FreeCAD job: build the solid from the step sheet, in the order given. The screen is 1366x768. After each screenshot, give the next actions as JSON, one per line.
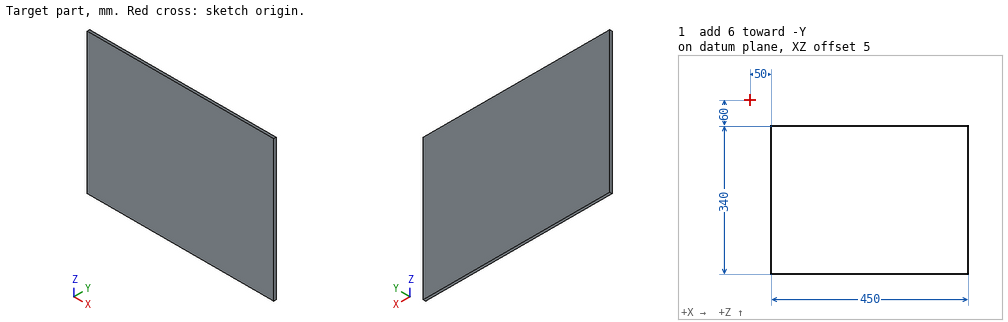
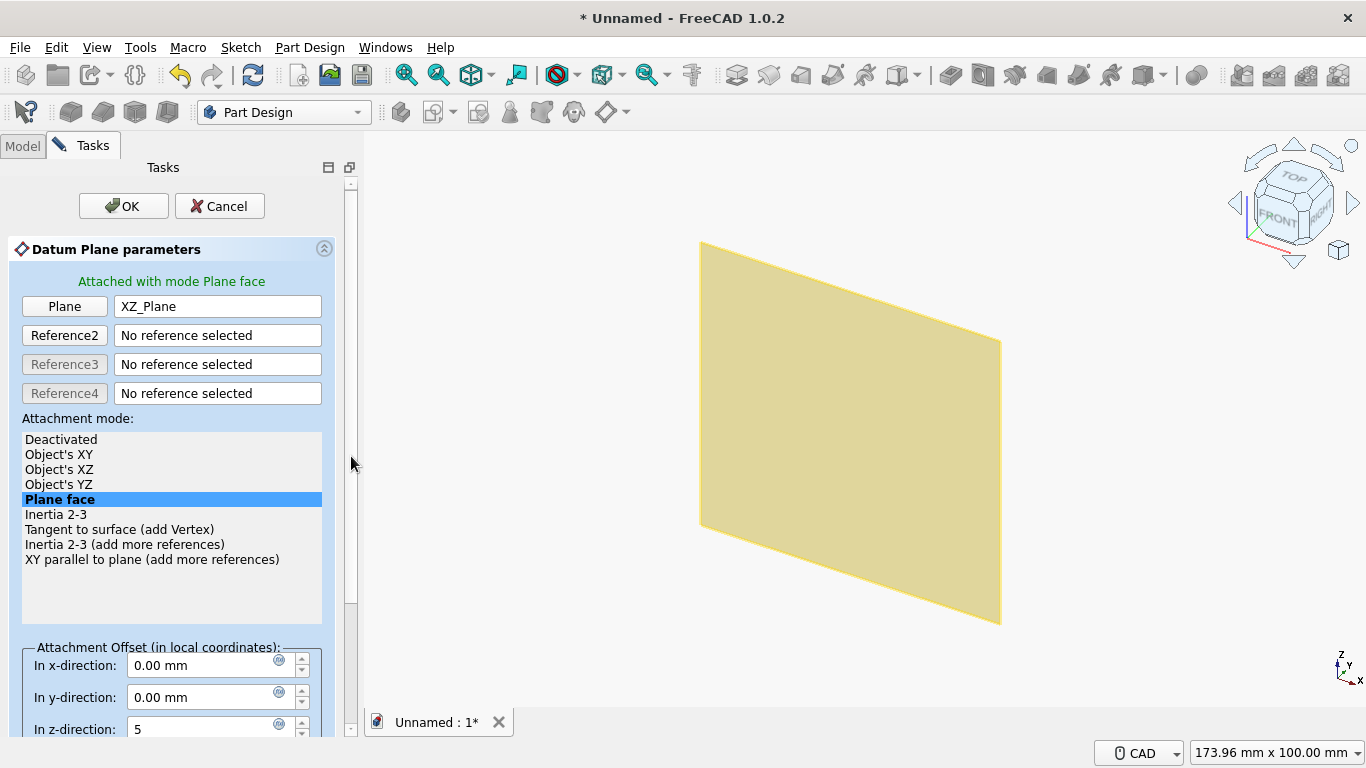
{"action": "left_click", "coordinate": [124, 206]}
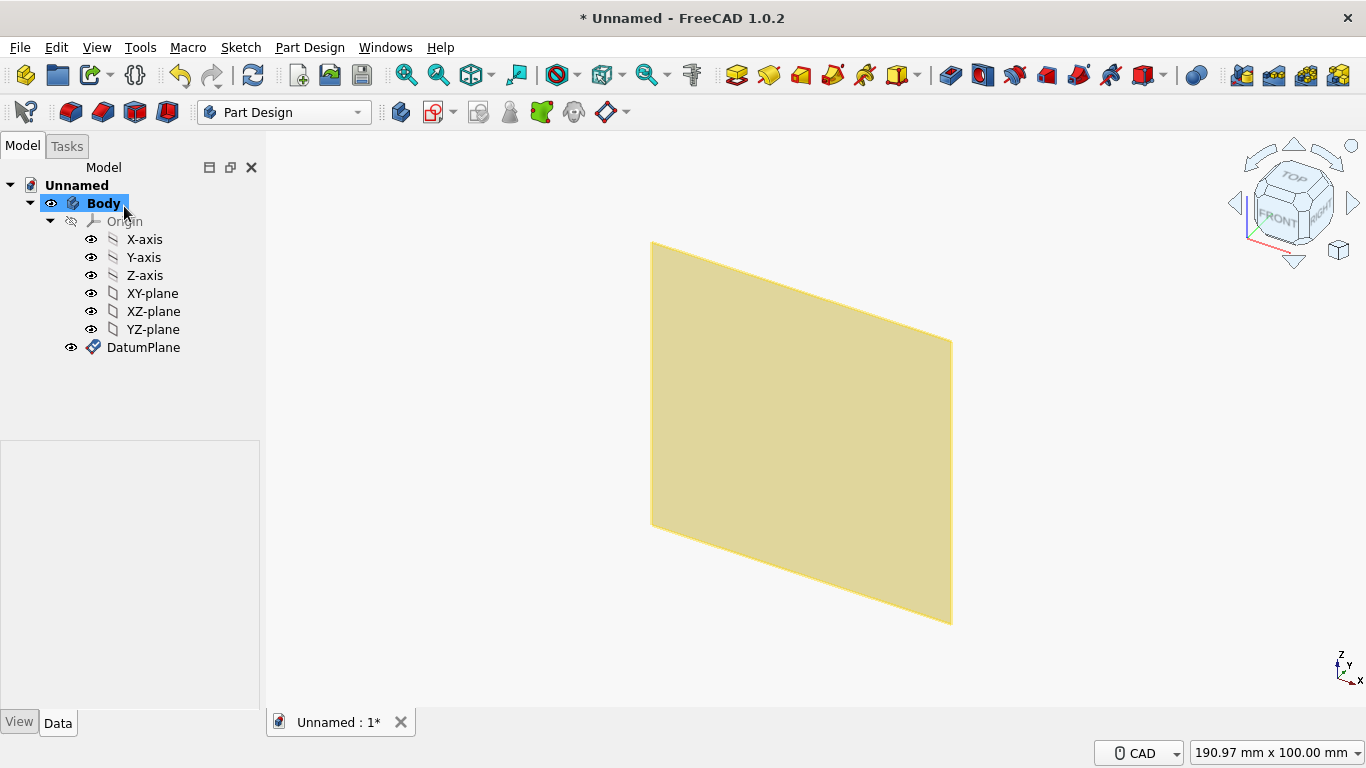
{"action": "left_click", "coordinate": [116, 347]}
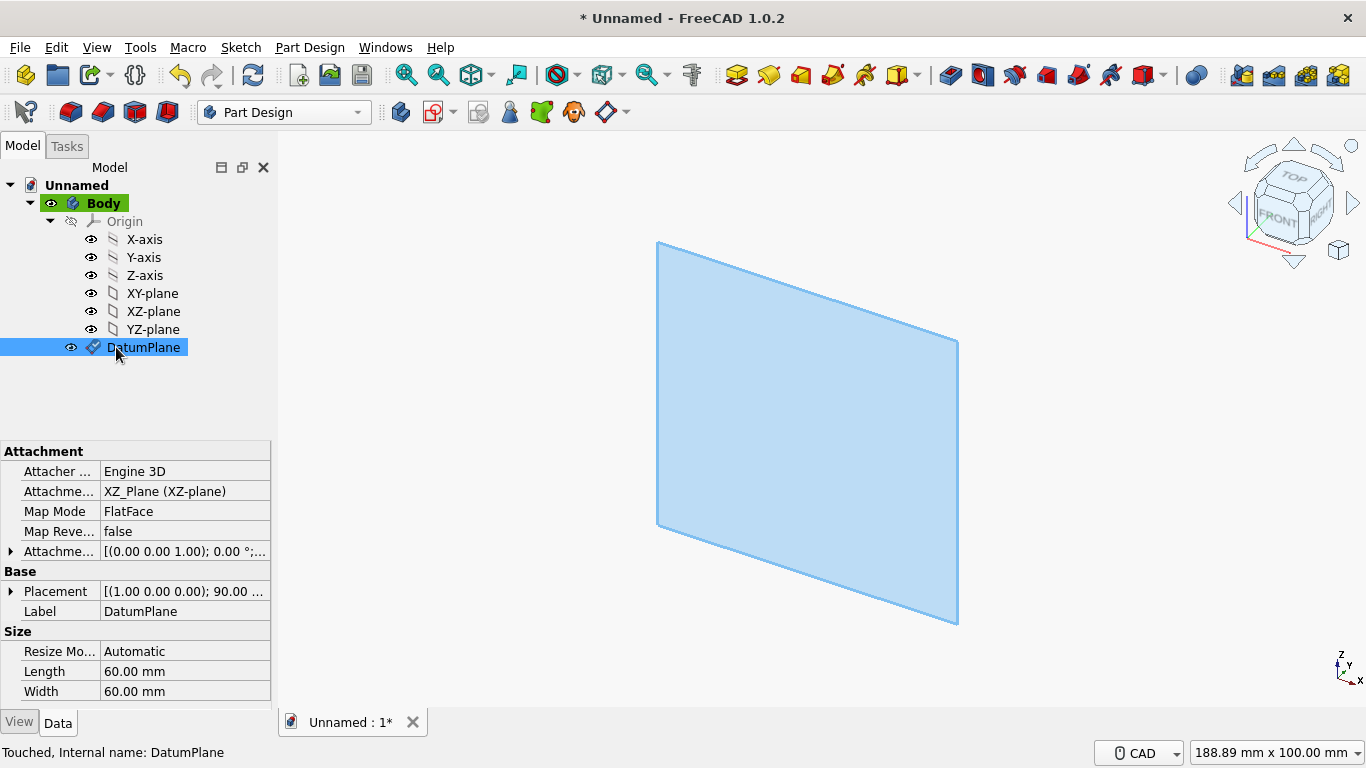
{"action": "left_click", "coordinate": [434, 112]}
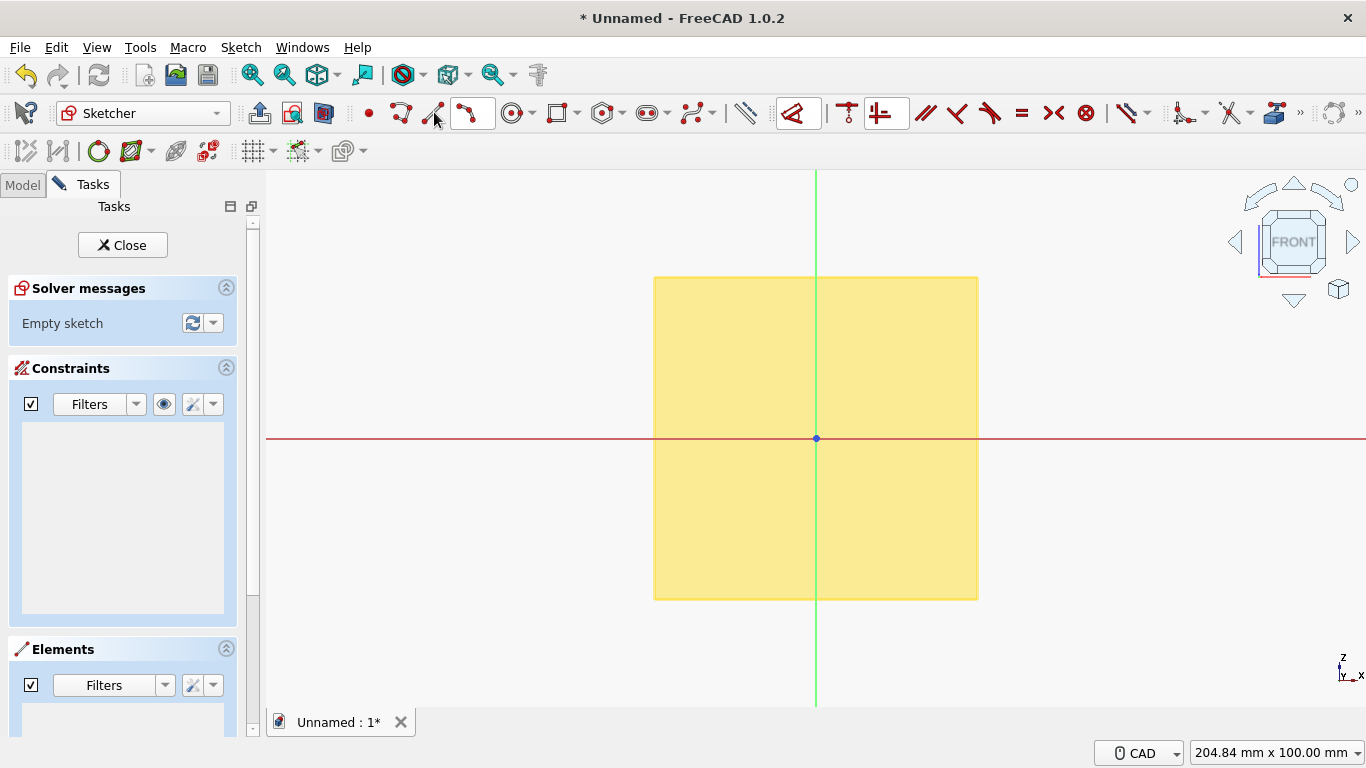
{"action": "scroll", "coordinate": [468, 226], "scroll_direction": "down", "scroll_amount": 9}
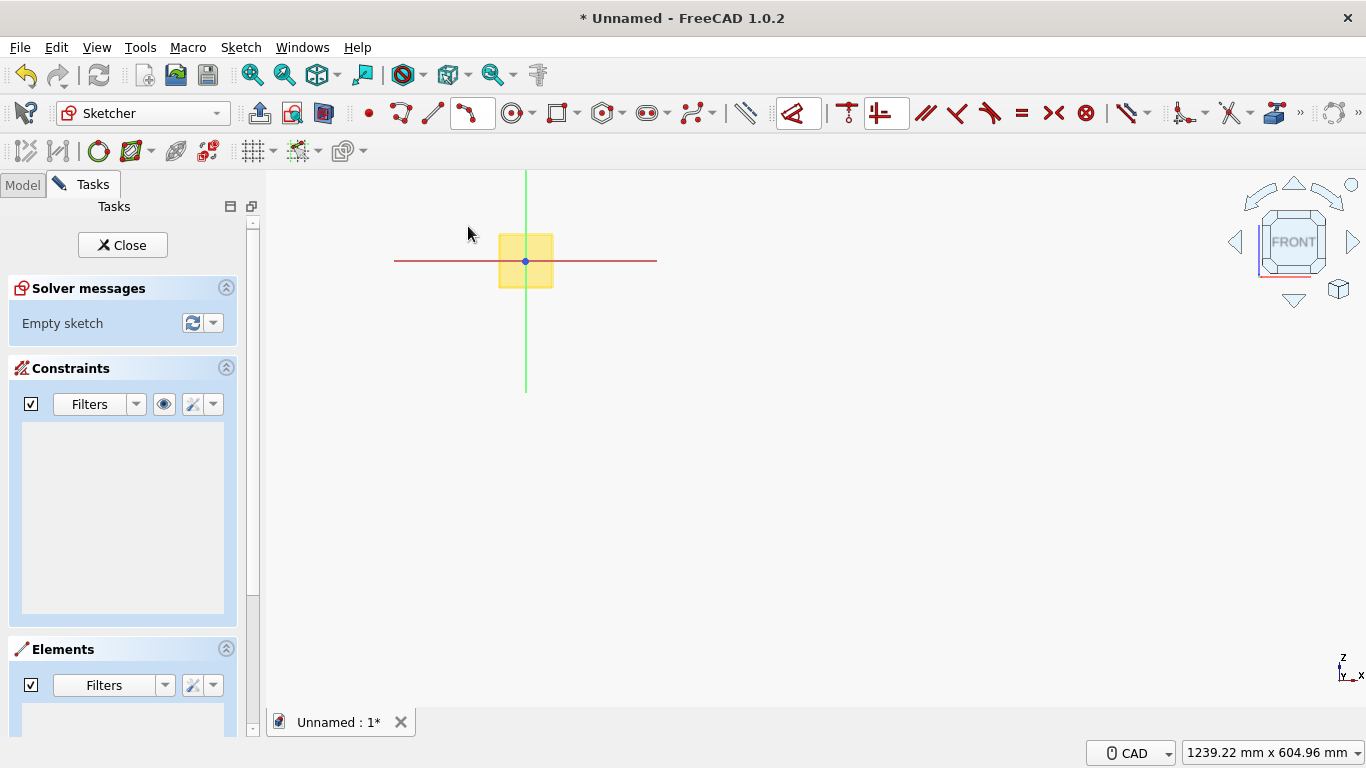
{"action": "key", "text": "g r"}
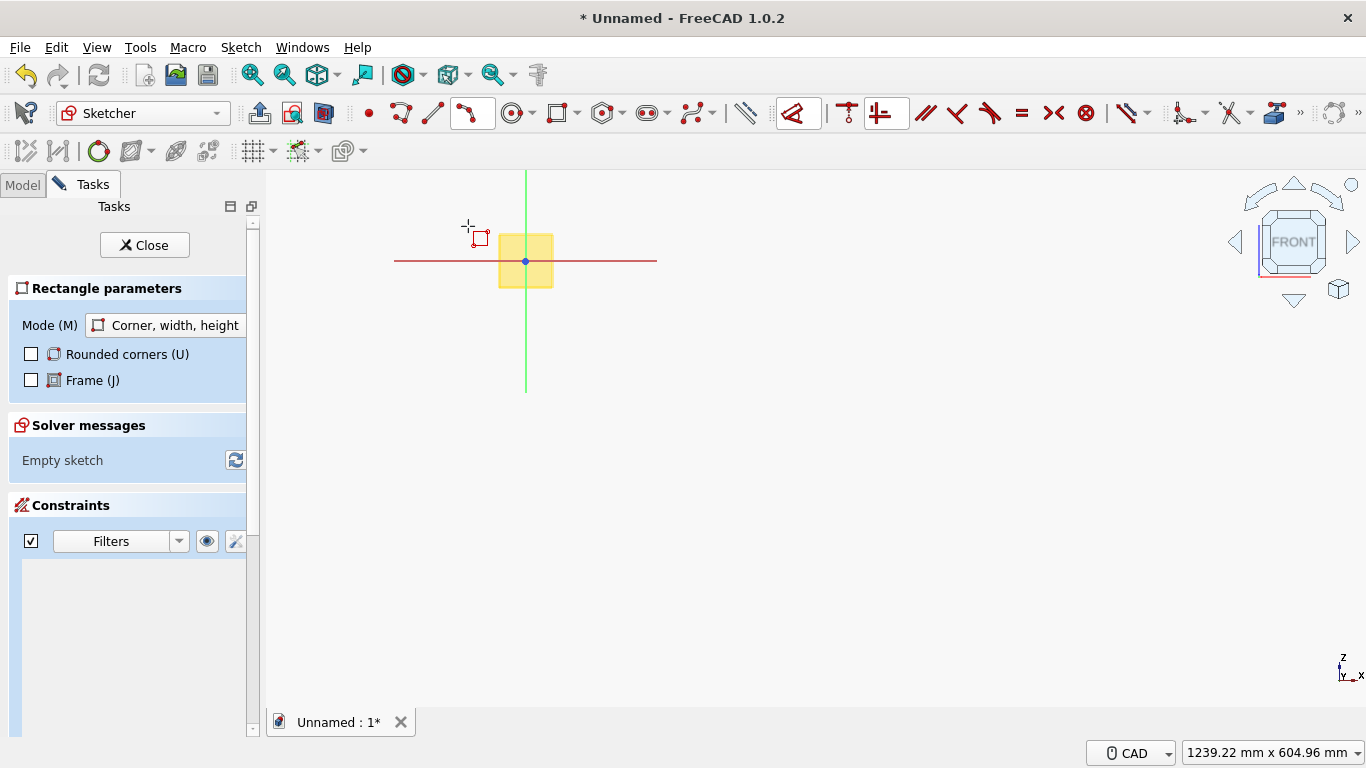
{"action": "left_click", "coordinate": [570, 314]}
{"action": "left_click", "coordinate": [970, 616]}
{"action": "key", "text": "Escape"}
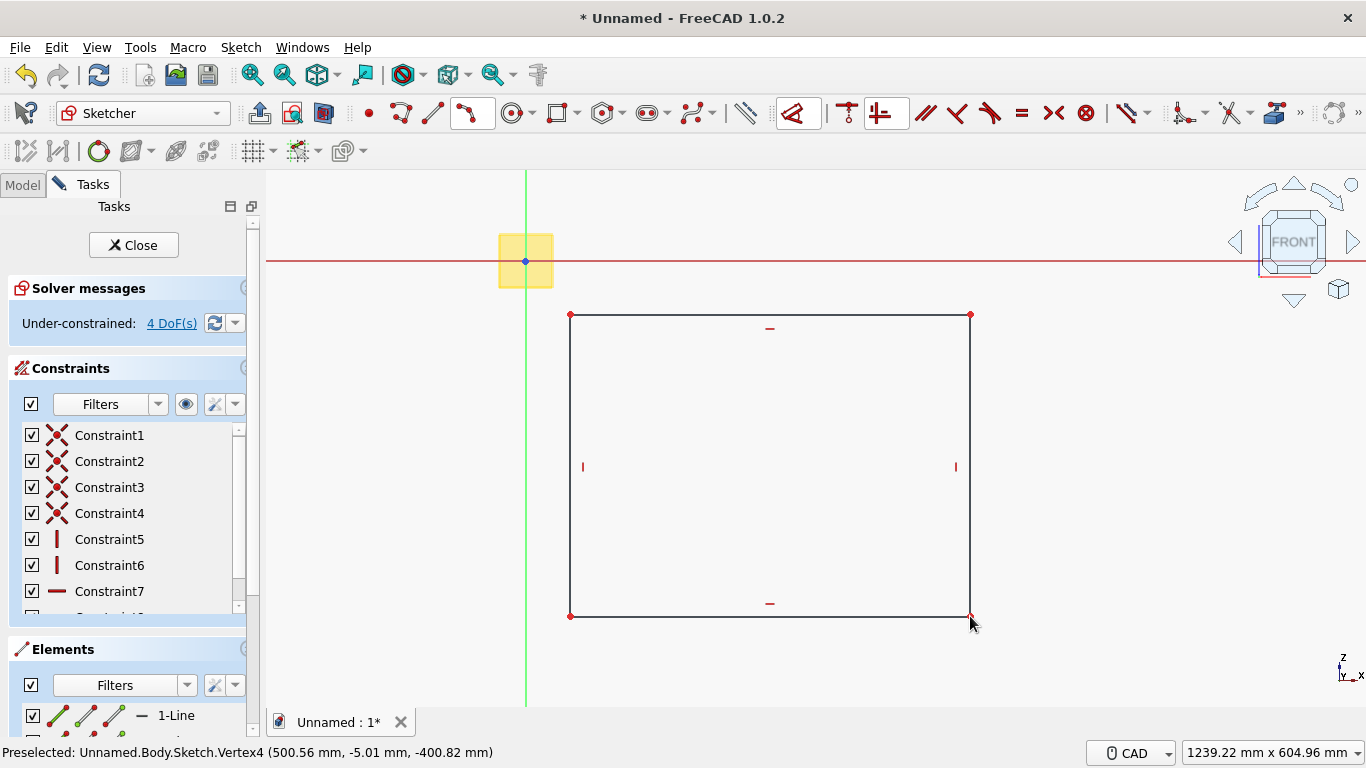
{"action": "key", "text": "d"}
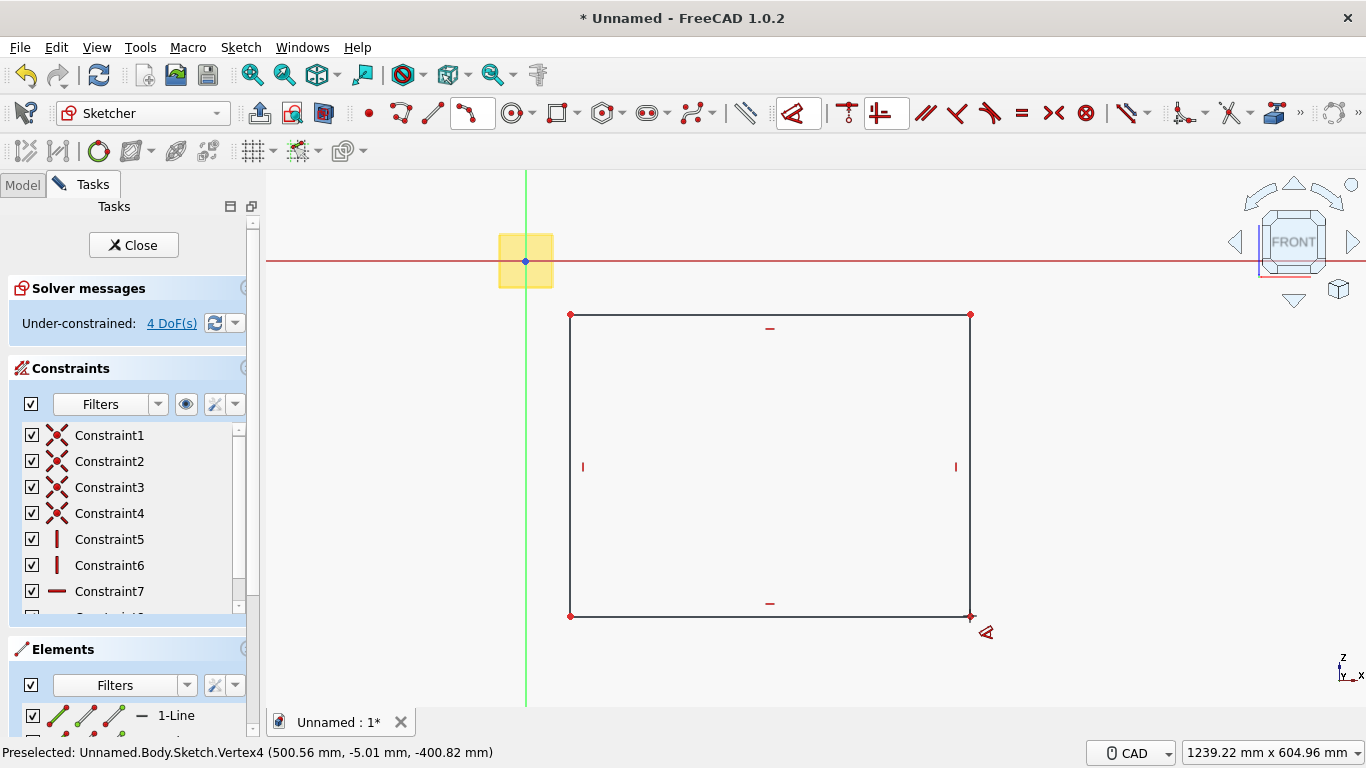
{"action": "left_click", "coordinate": [570, 406]}
{"action": "left_click", "coordinate": [604, 466]}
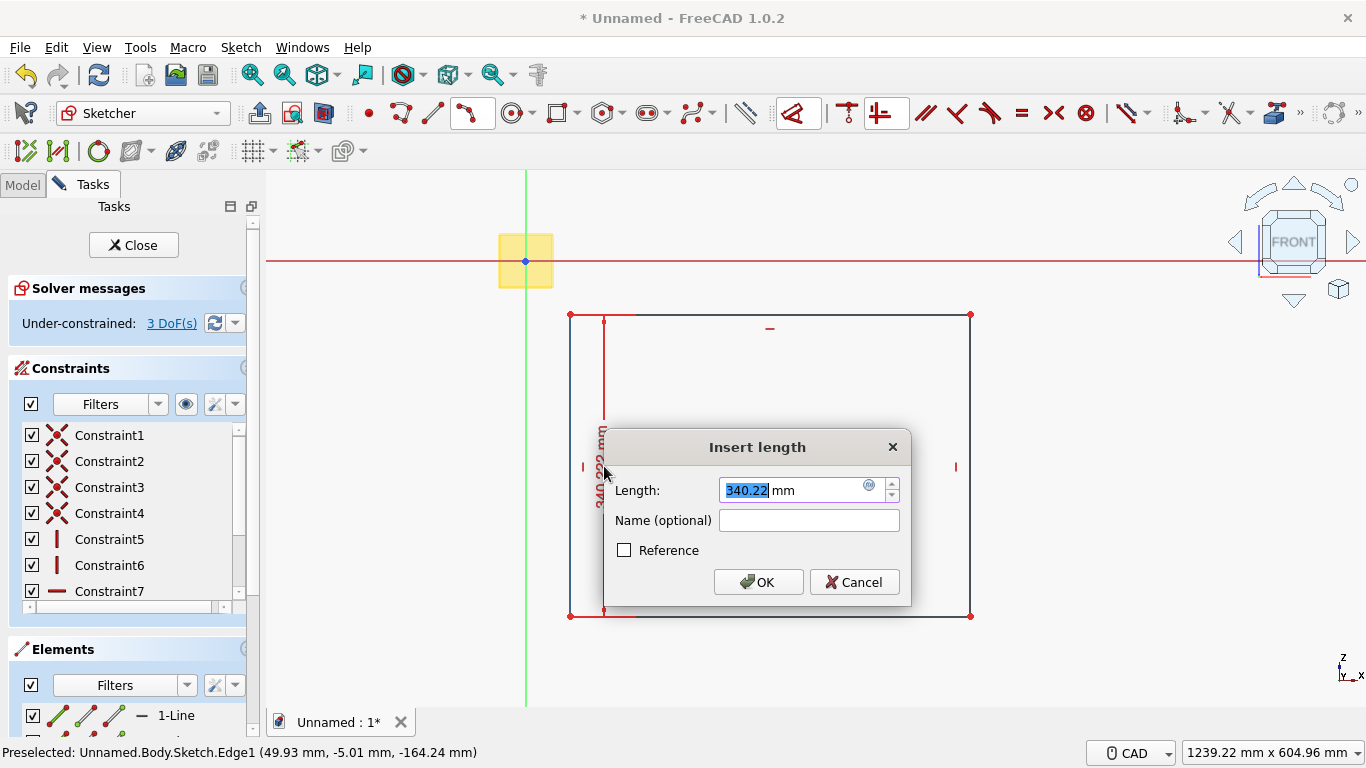
{"action": "type", "text": "340"}
{"action": "key", "text": "Return"}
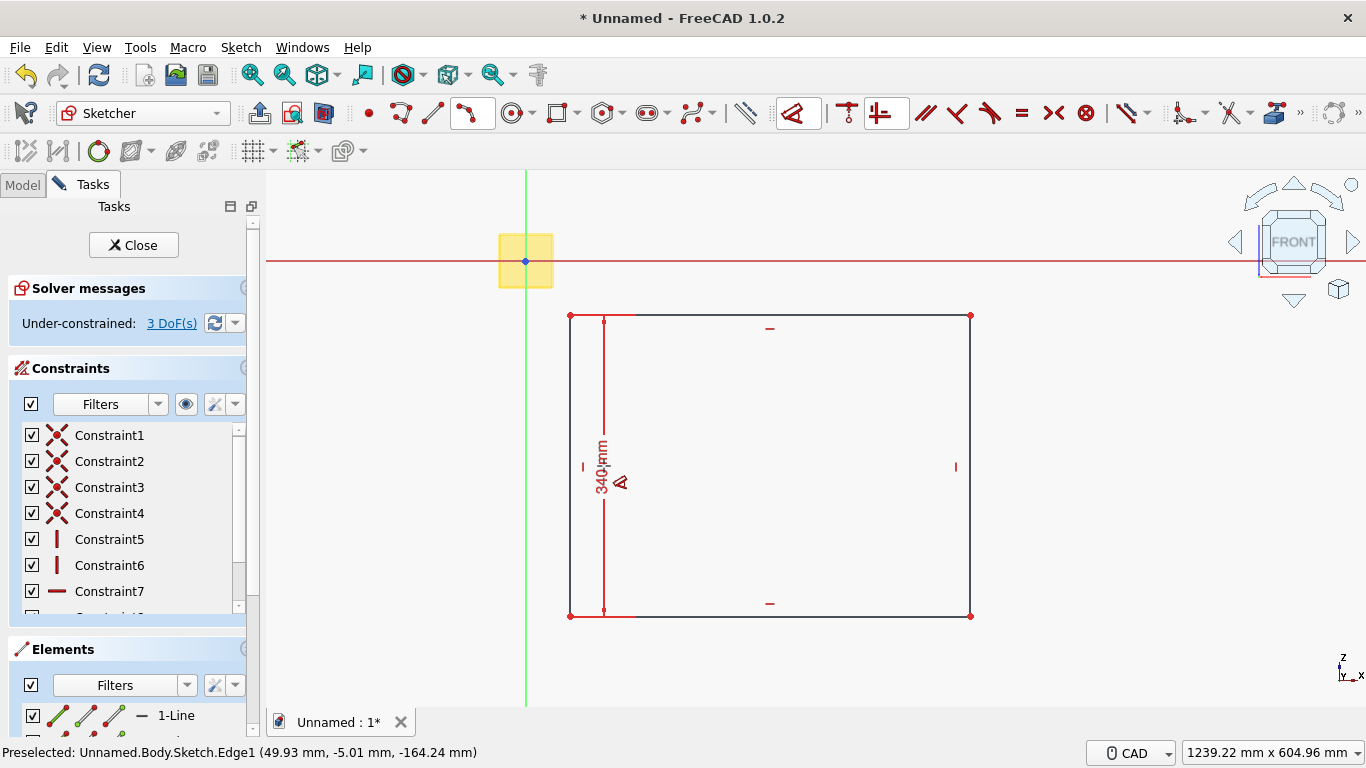
{"action": "left_click", "coordinate": [690, 617]}
{"action": "left_click", "coordinate": [770, 651]}